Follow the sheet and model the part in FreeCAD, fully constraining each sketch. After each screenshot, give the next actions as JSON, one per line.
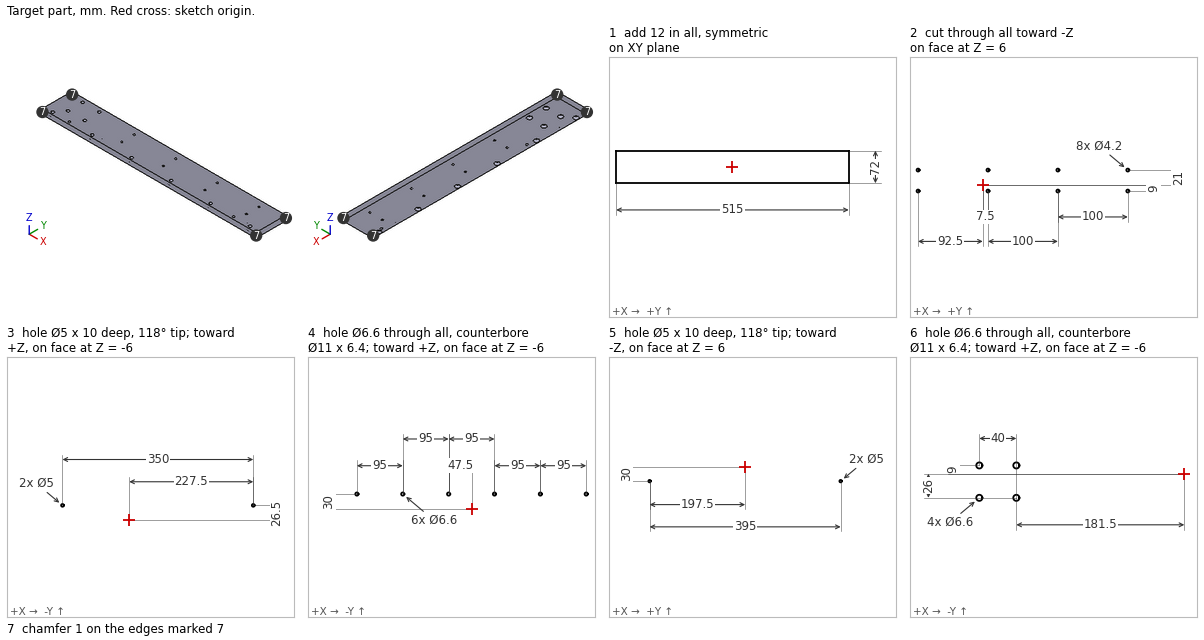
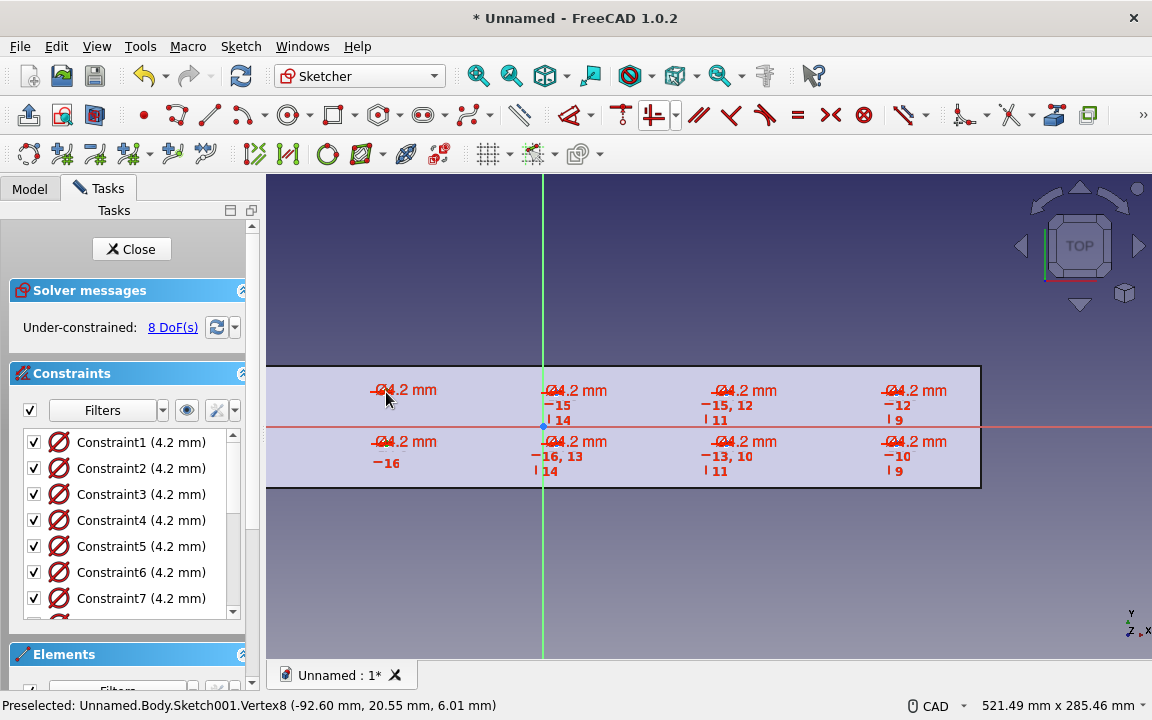
{"action": "left_click", "coordinate": [676, 116]}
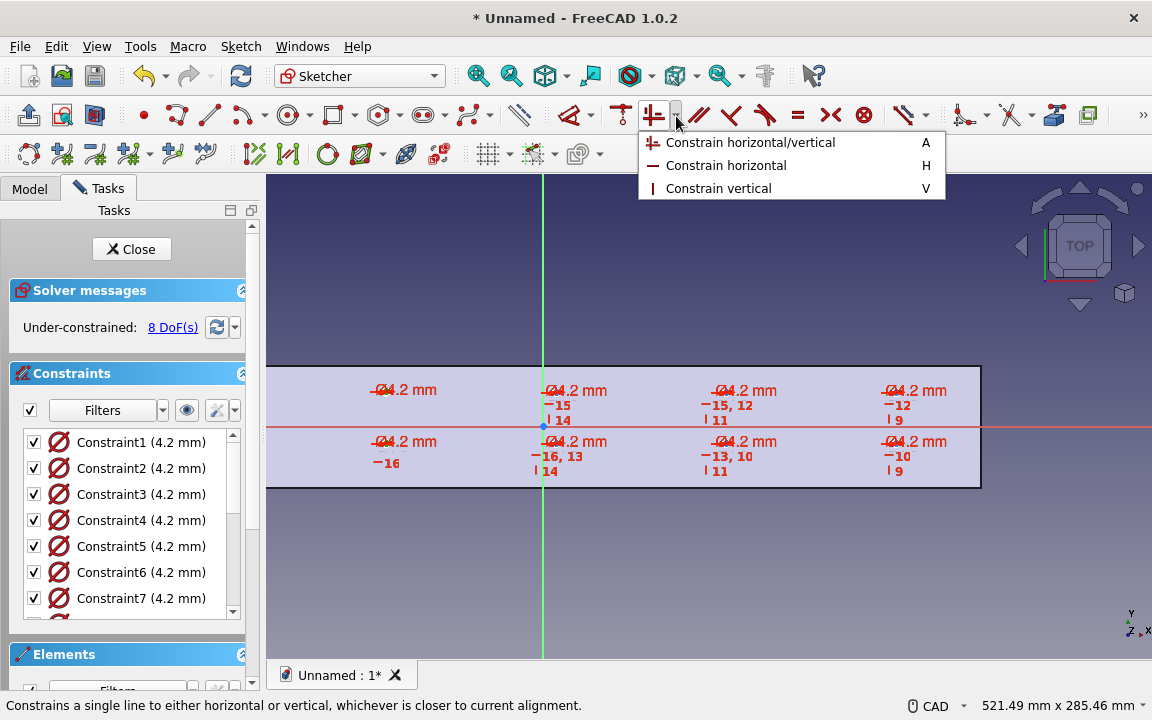
{"action": "left_click", "coordinate": [792, 188]}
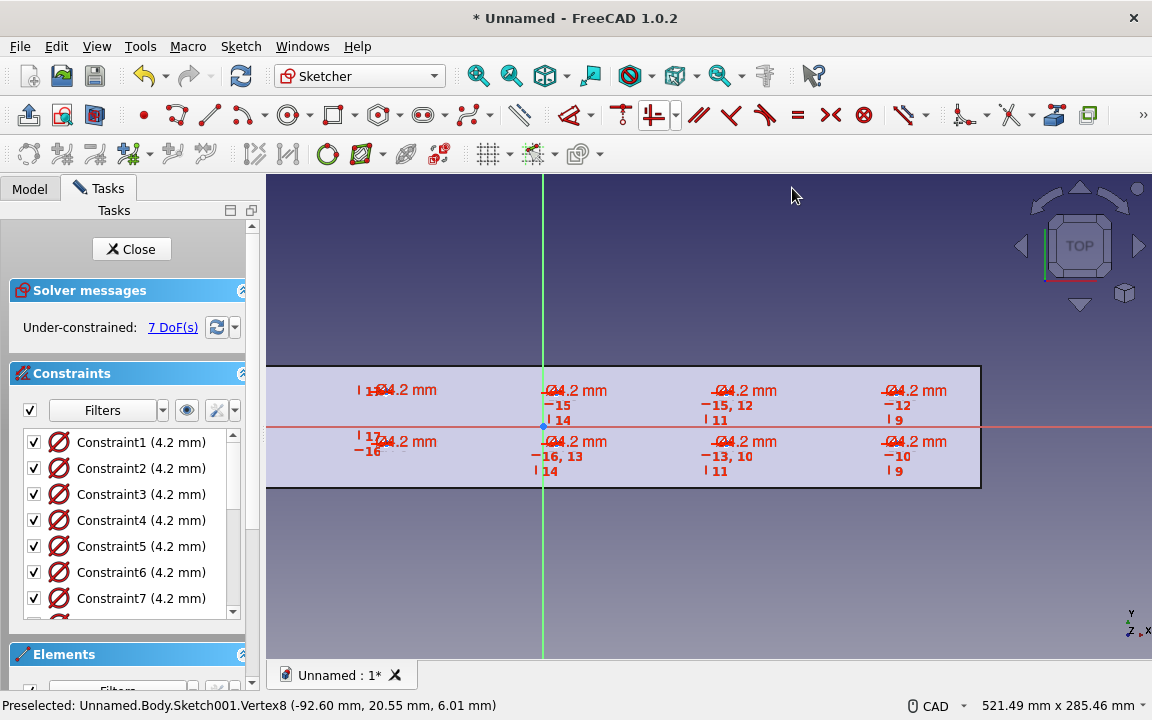
{"action": "left_click", "coordinate": [556, 393]}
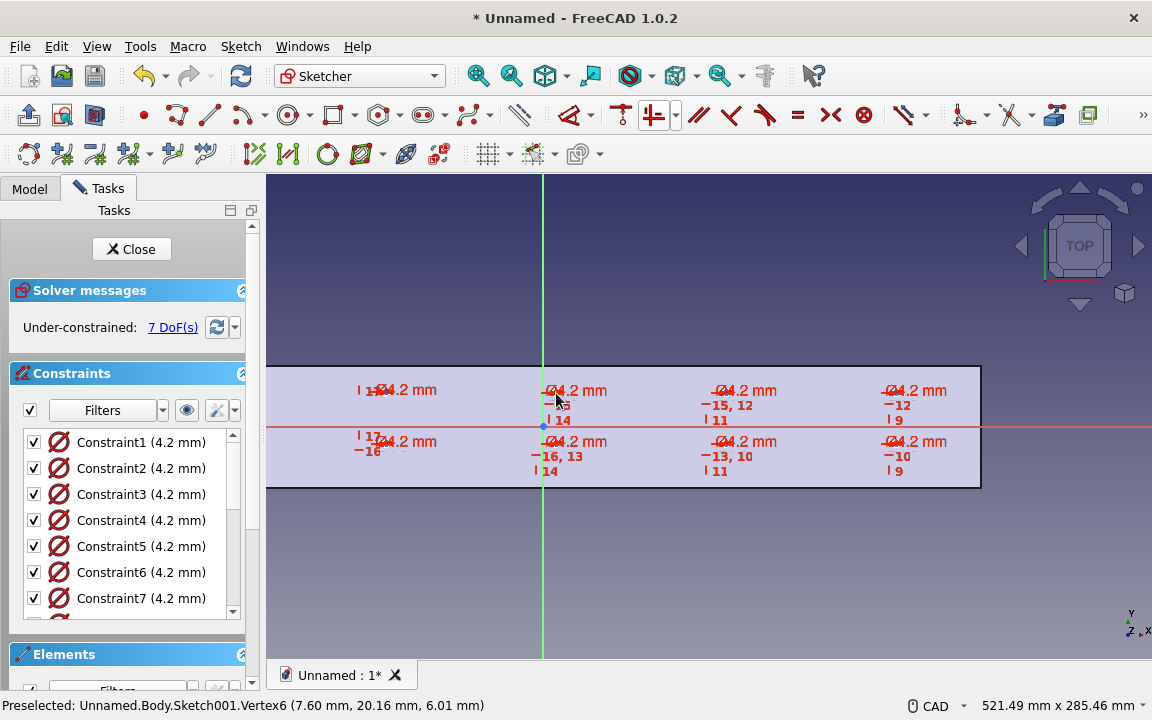
{"action": "left_click", "coordinate": [386, 392]}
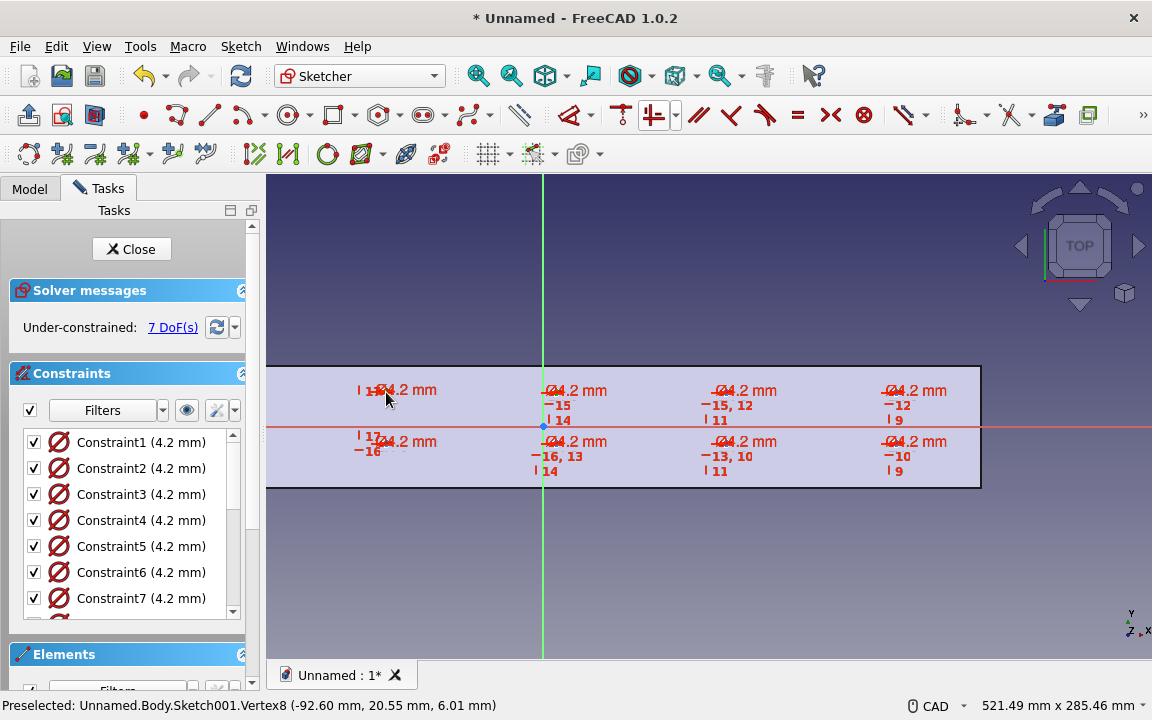
{"action": "key", "text": "h"}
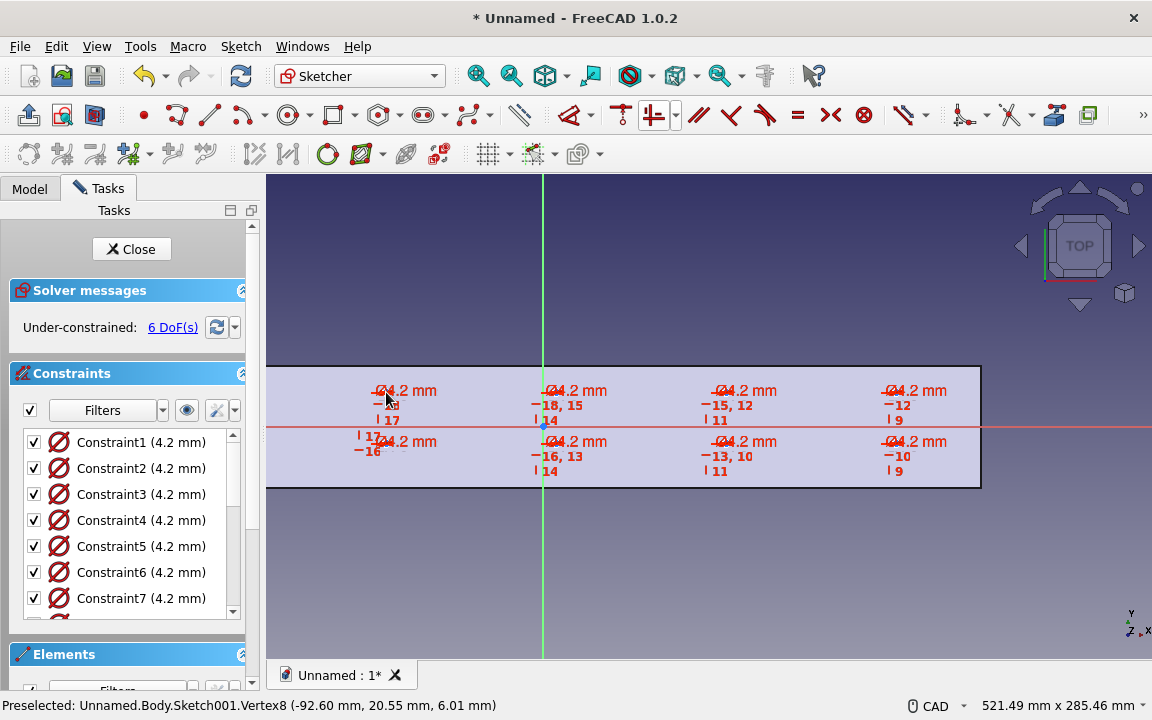
{"action": "scroll", "coordinate": [896, 444], "scroll_direction": "up", "scroll_amount": 5}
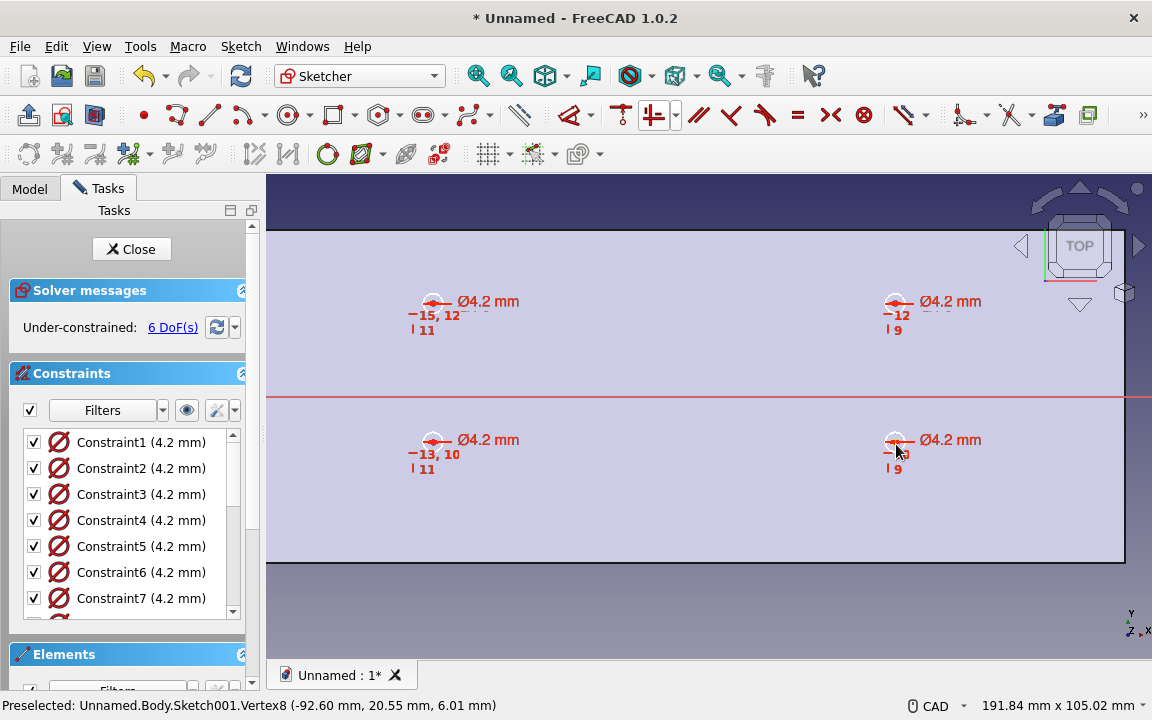
{"action": "left_click", "coordinate": [895, 442]}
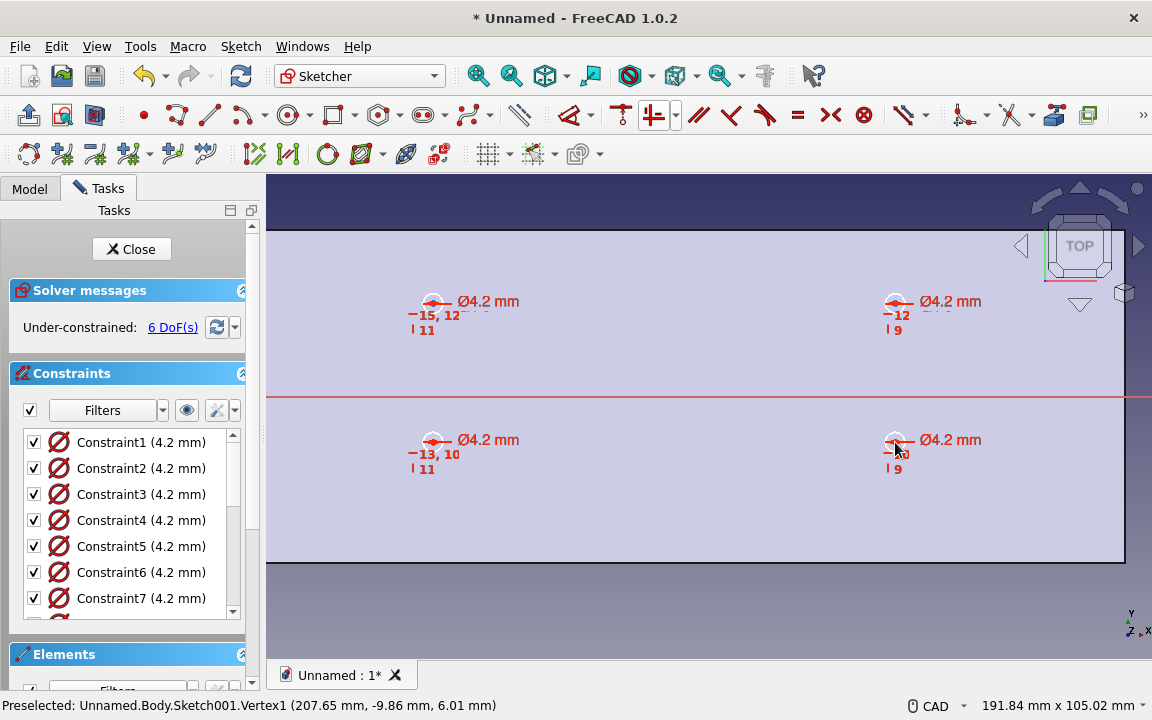
{"action": "left_click", "coordinate": [590, 116]}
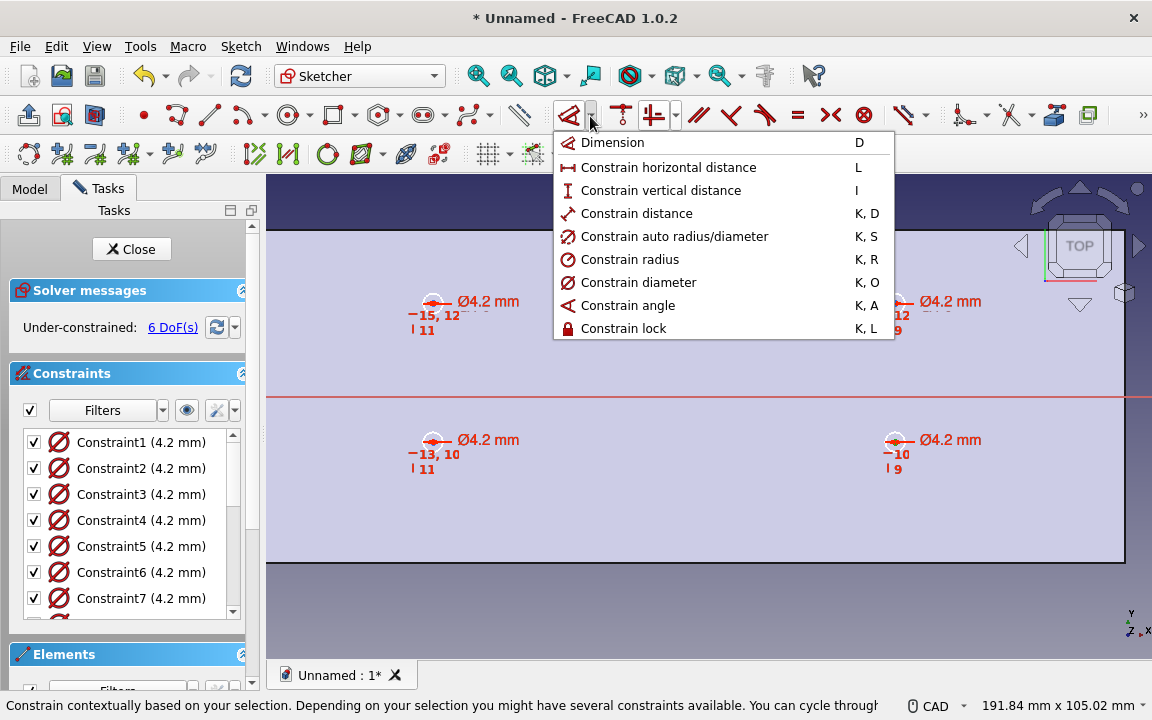
{"action": "left_click", "coordinate": [724, 190]}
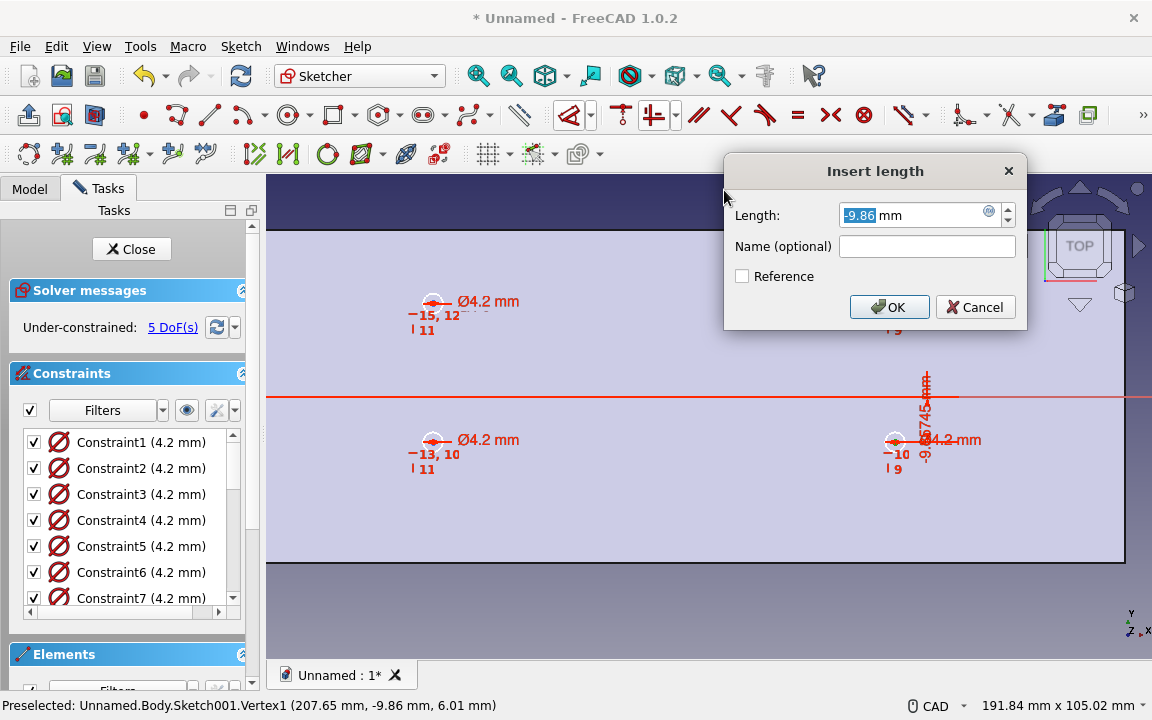
{"action": "type", "text": "-9"}
{"action": "key", "text": "Return"}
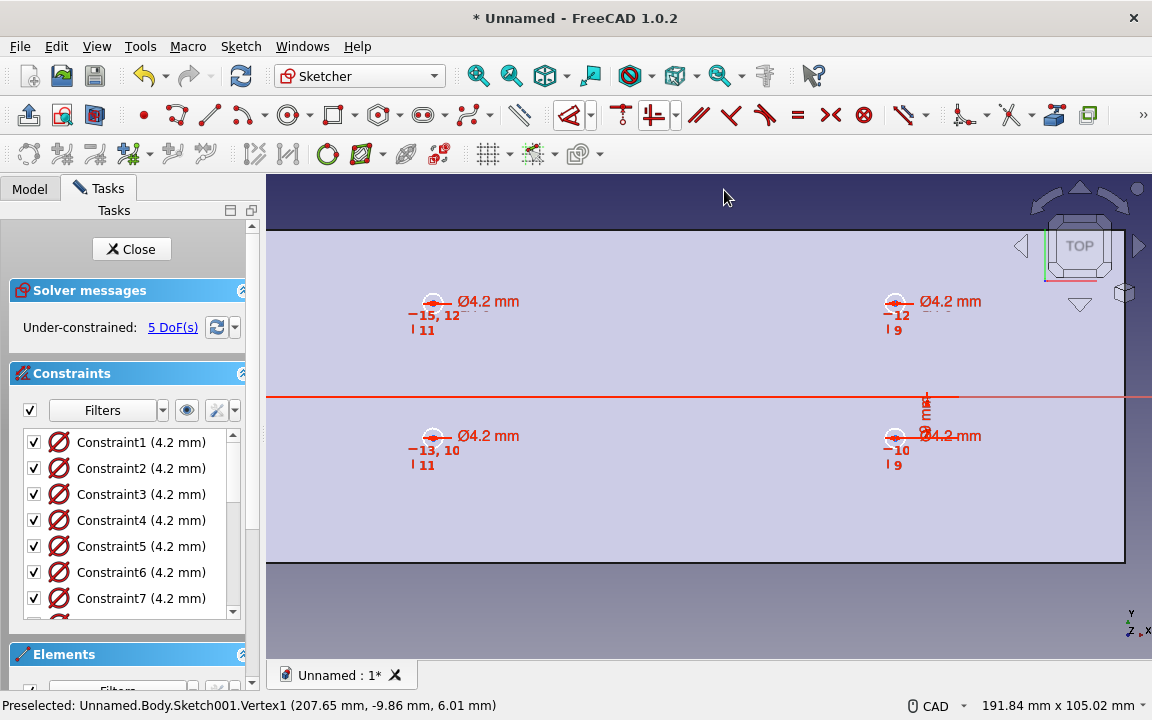
{"action": "left_click", "coordinate": [895, 304]}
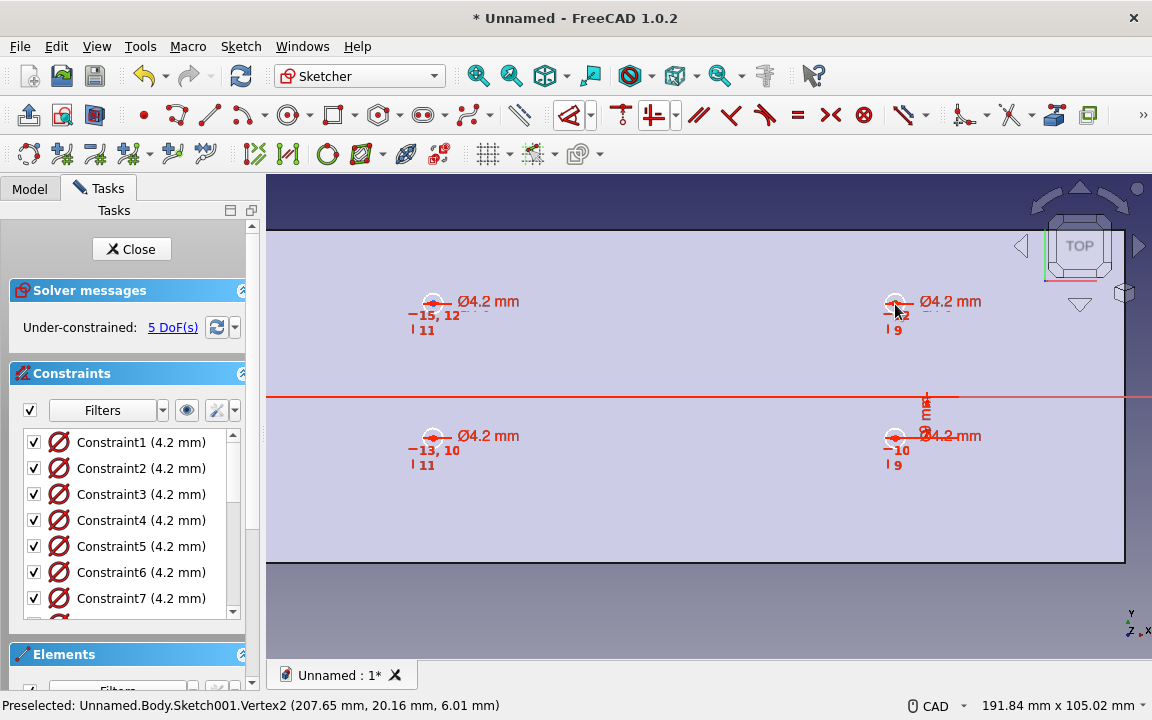
{"action": "key", "text": "i"}